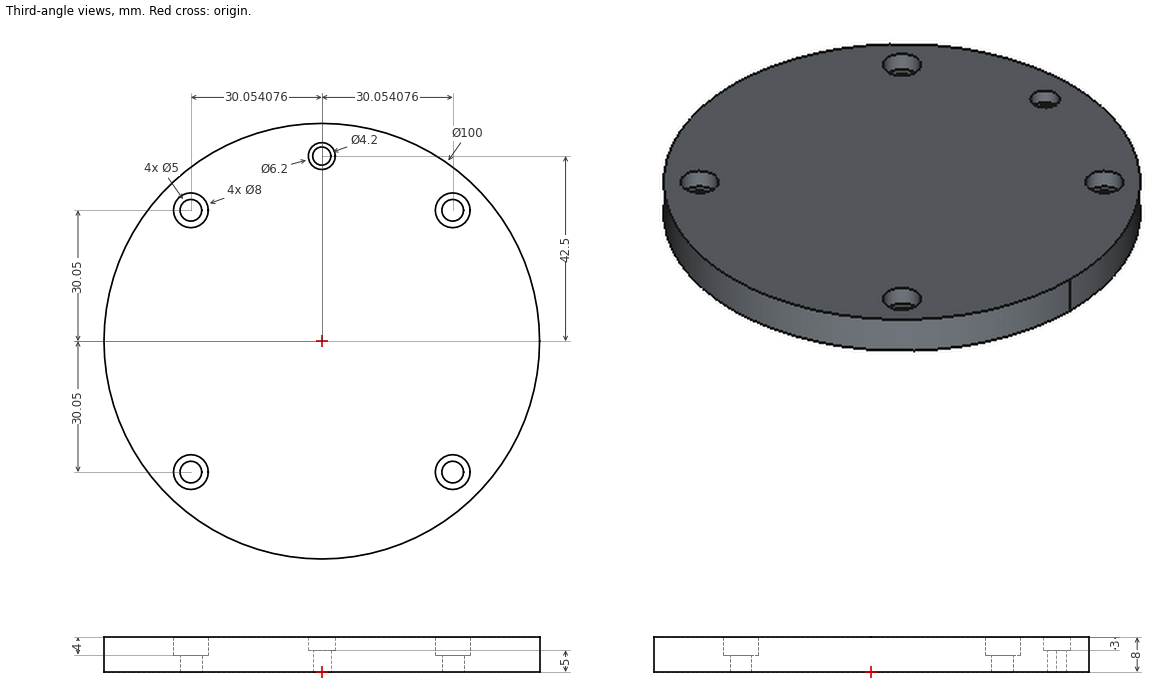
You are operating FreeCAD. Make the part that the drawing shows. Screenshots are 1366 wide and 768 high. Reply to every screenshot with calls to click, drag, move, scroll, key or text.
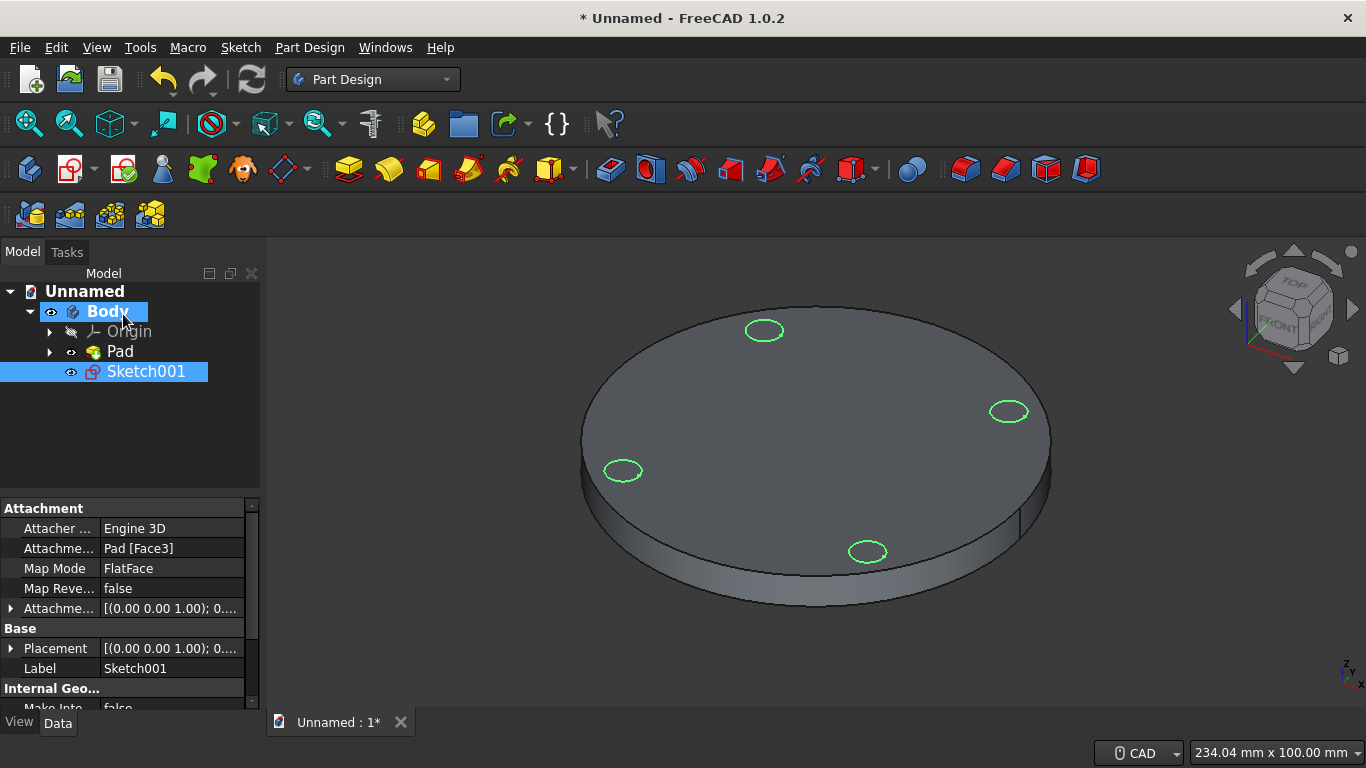
click(612, 170)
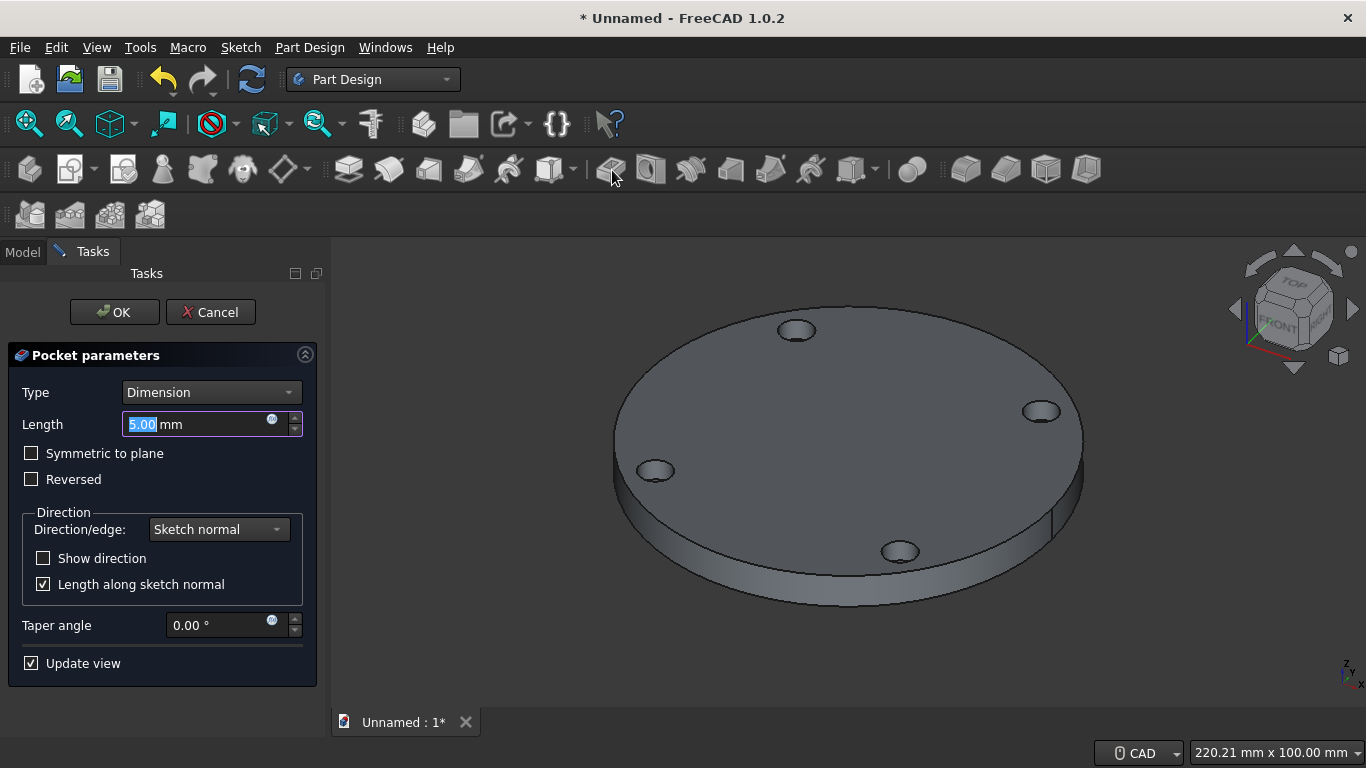
text(4)
key(Tab)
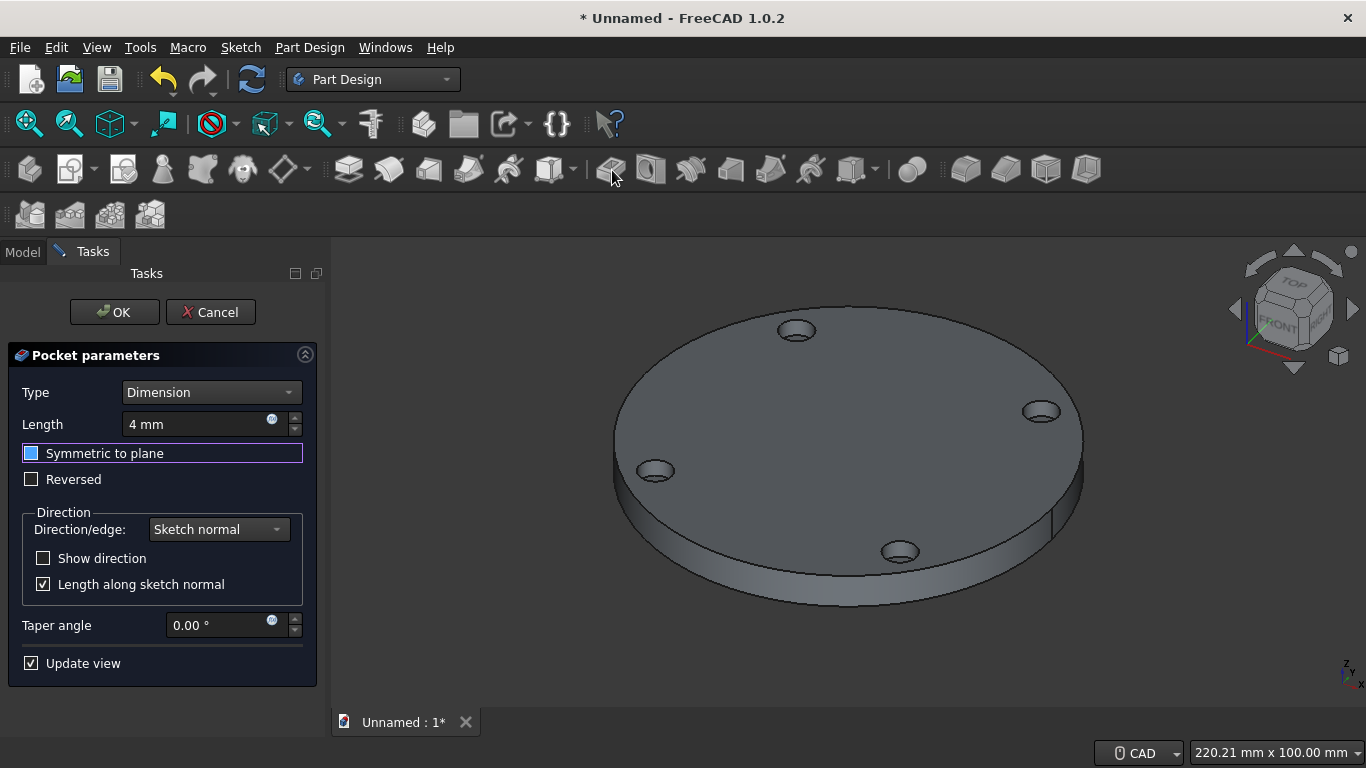
click(115, 312)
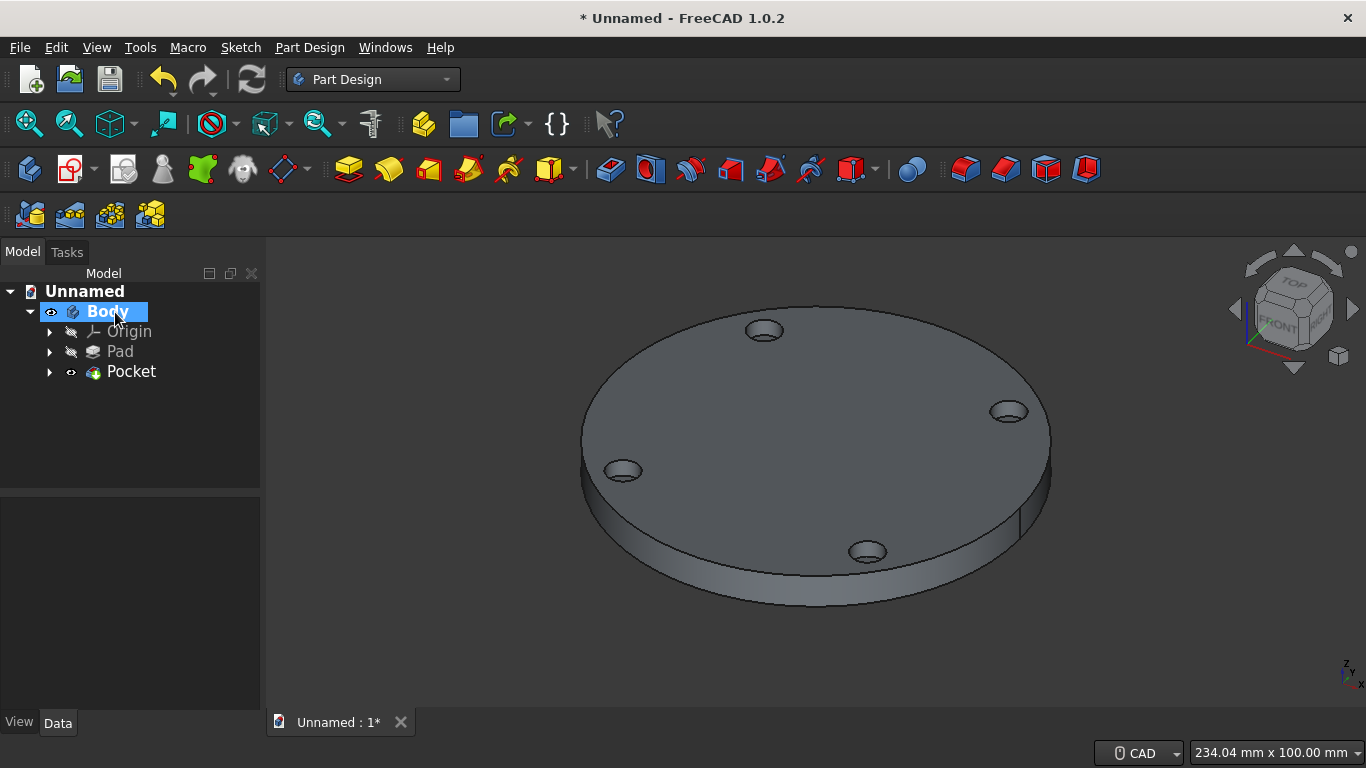
click(816, 440)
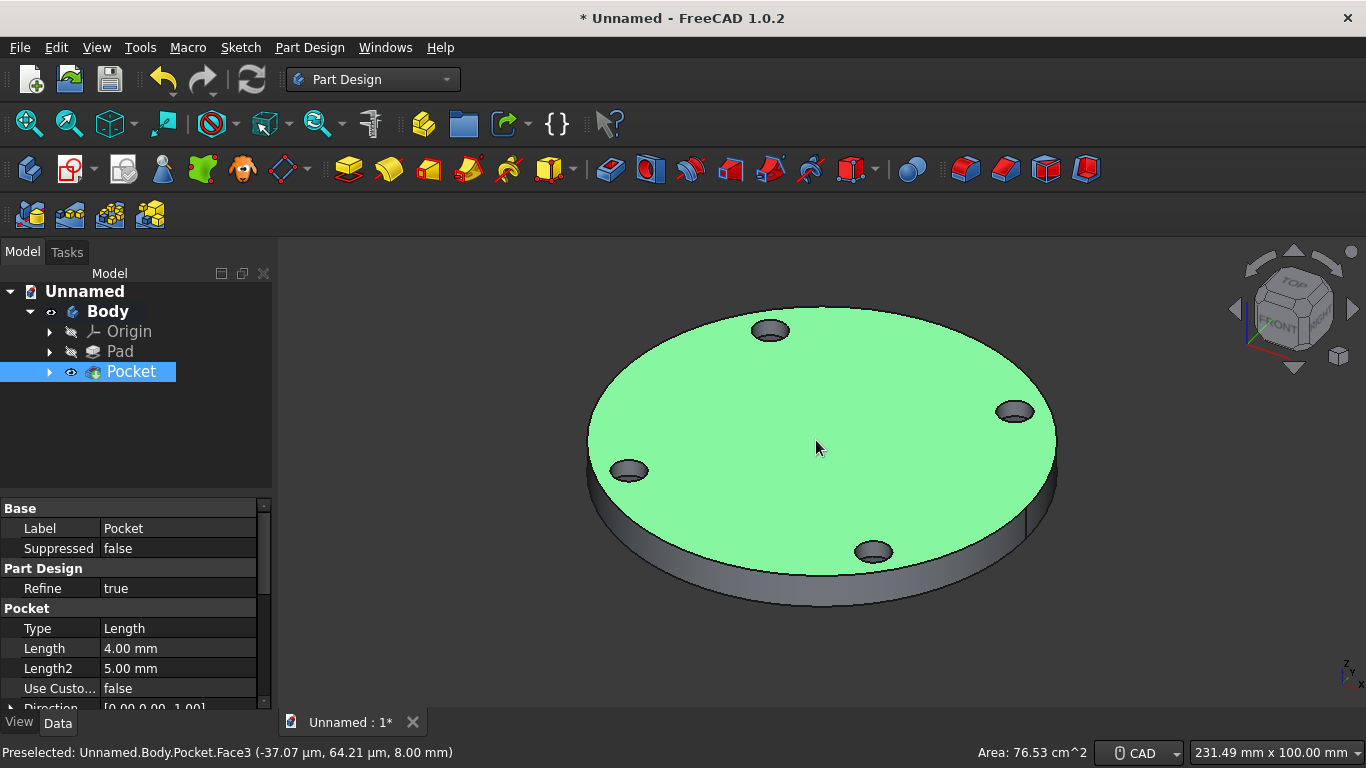
click(70, 170)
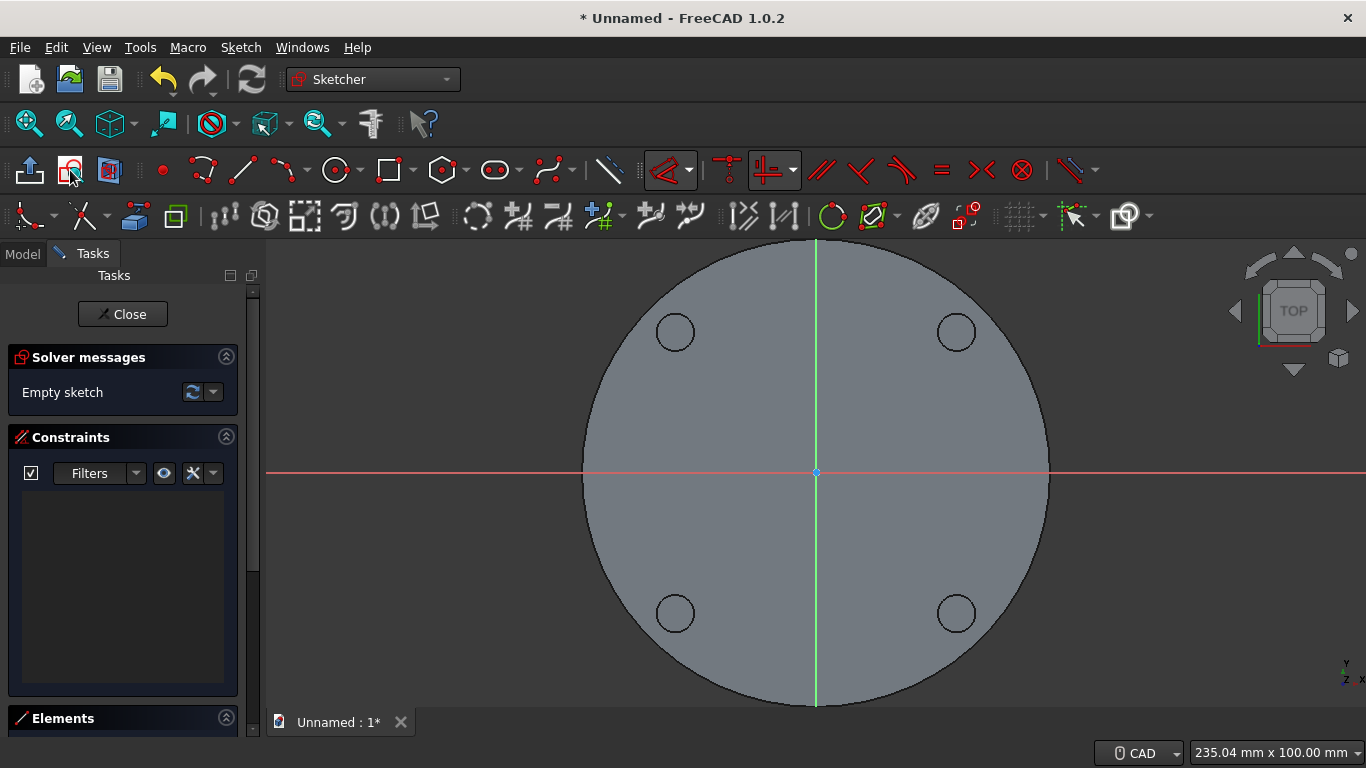
scroll(748, 473, down, 5)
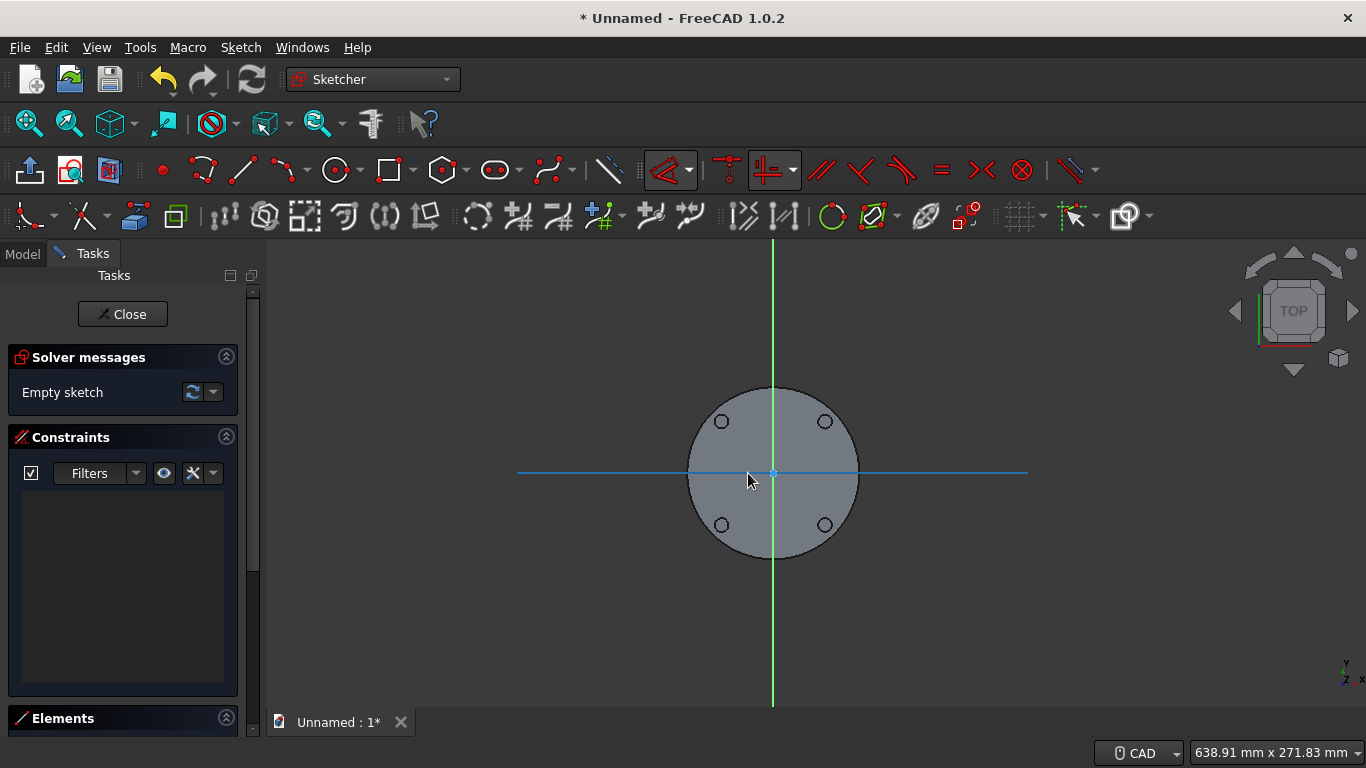
scroll(775, 396, up, 15)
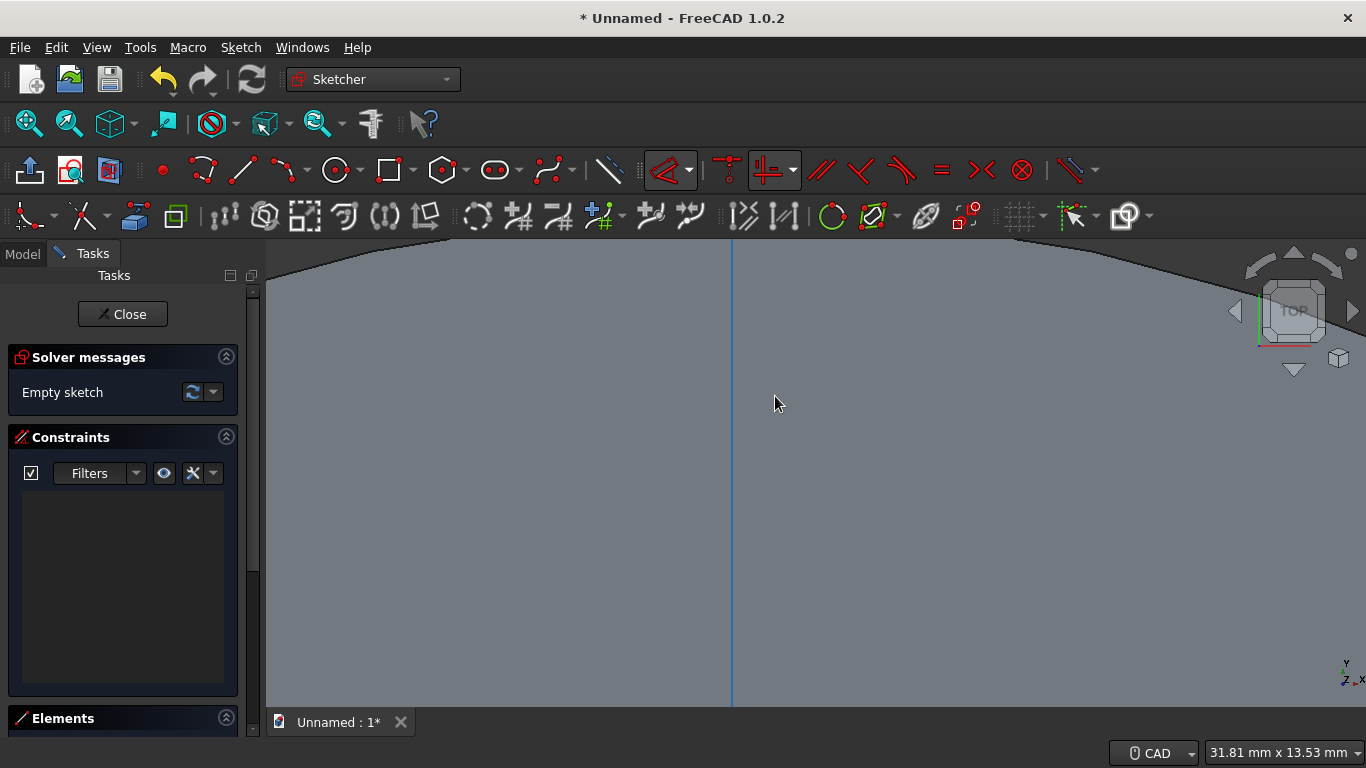
scroll(700, 473, up, 2)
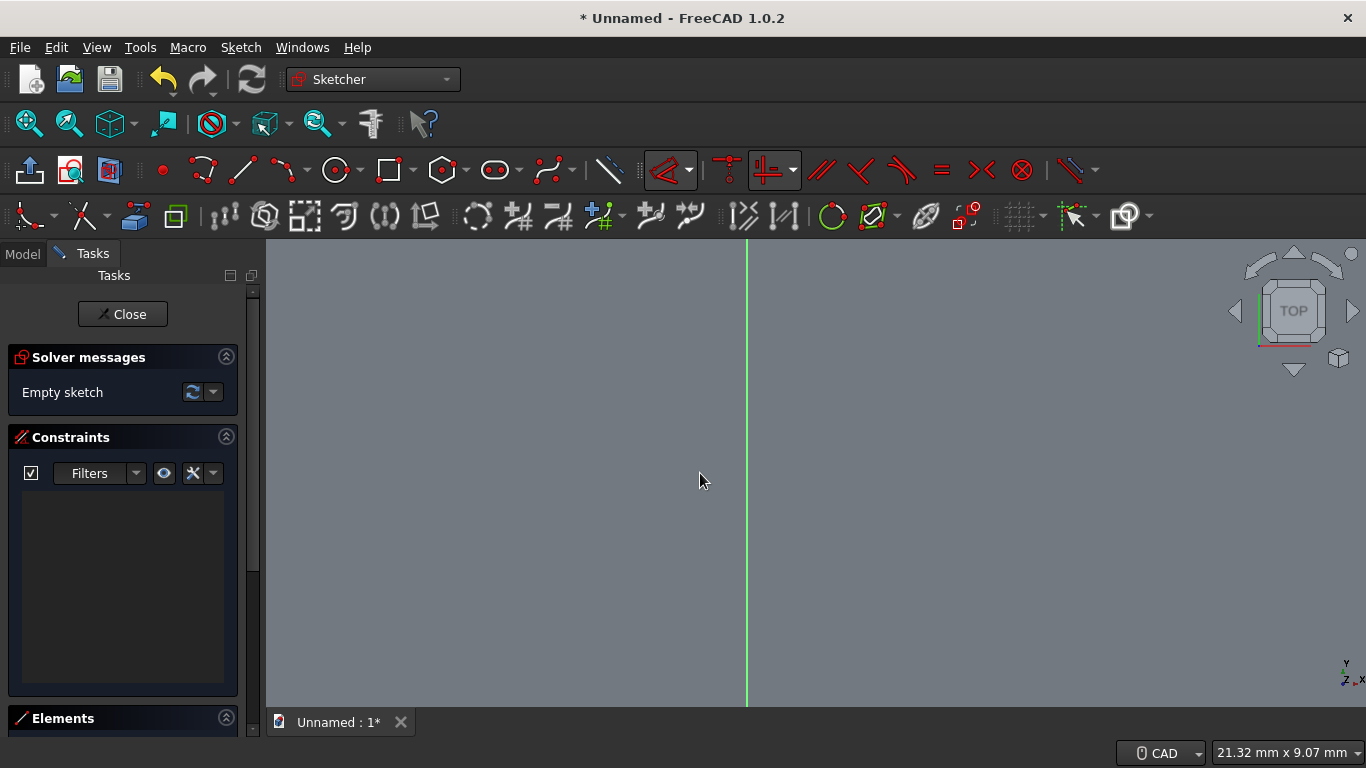
click(336, 170)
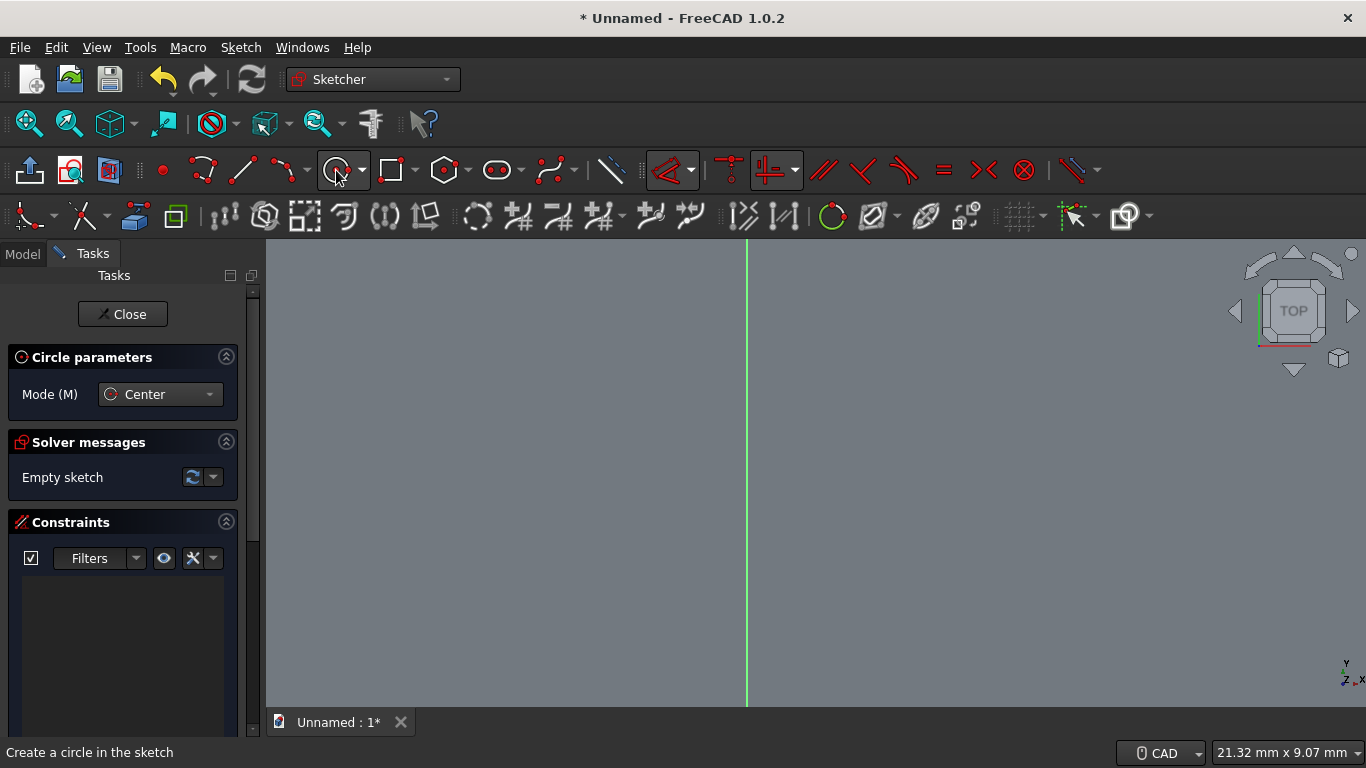
click(747, 473)
move(860, 359)